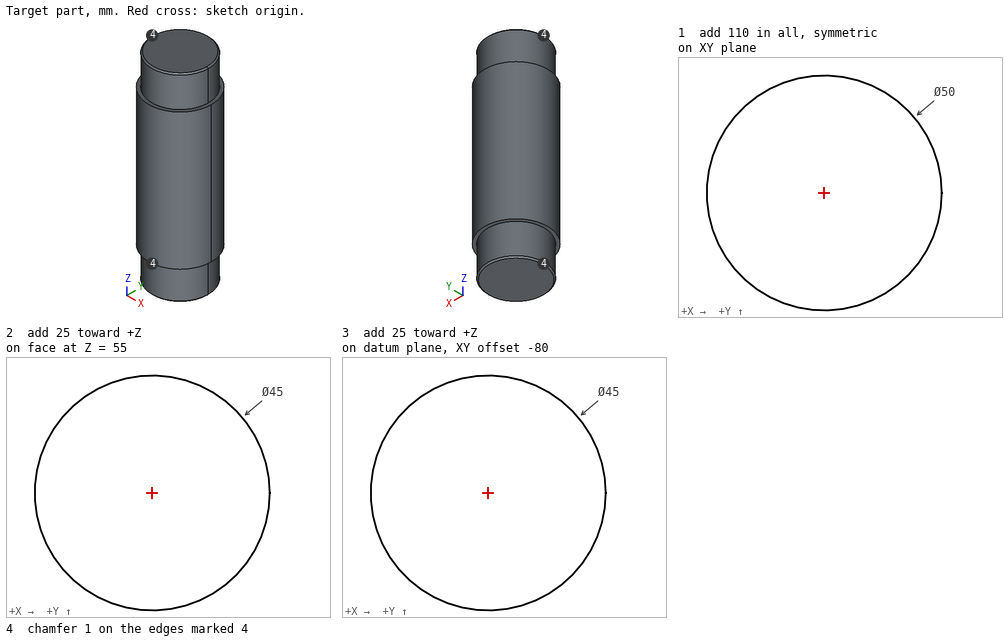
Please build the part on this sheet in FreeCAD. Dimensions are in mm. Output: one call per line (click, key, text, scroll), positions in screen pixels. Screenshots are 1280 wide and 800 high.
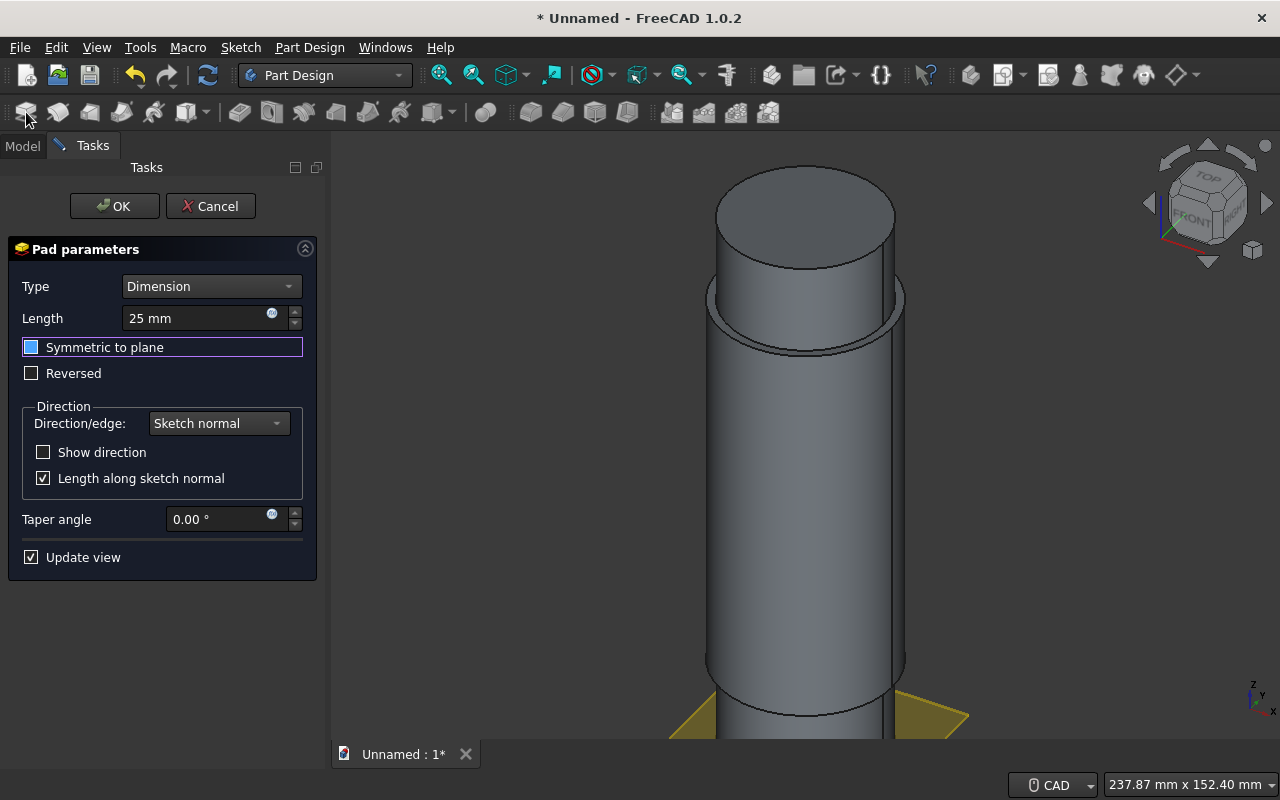
click(115, 206)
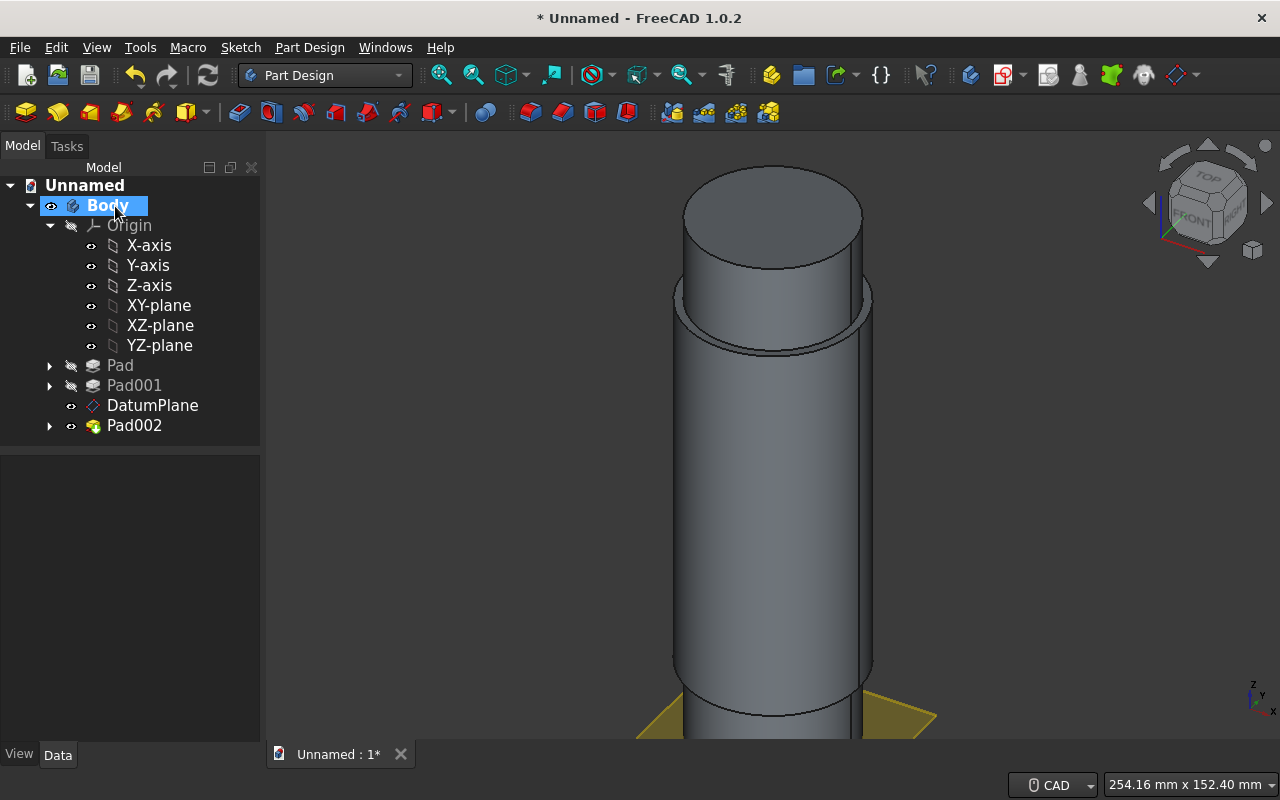
click(116, 406)
key(space)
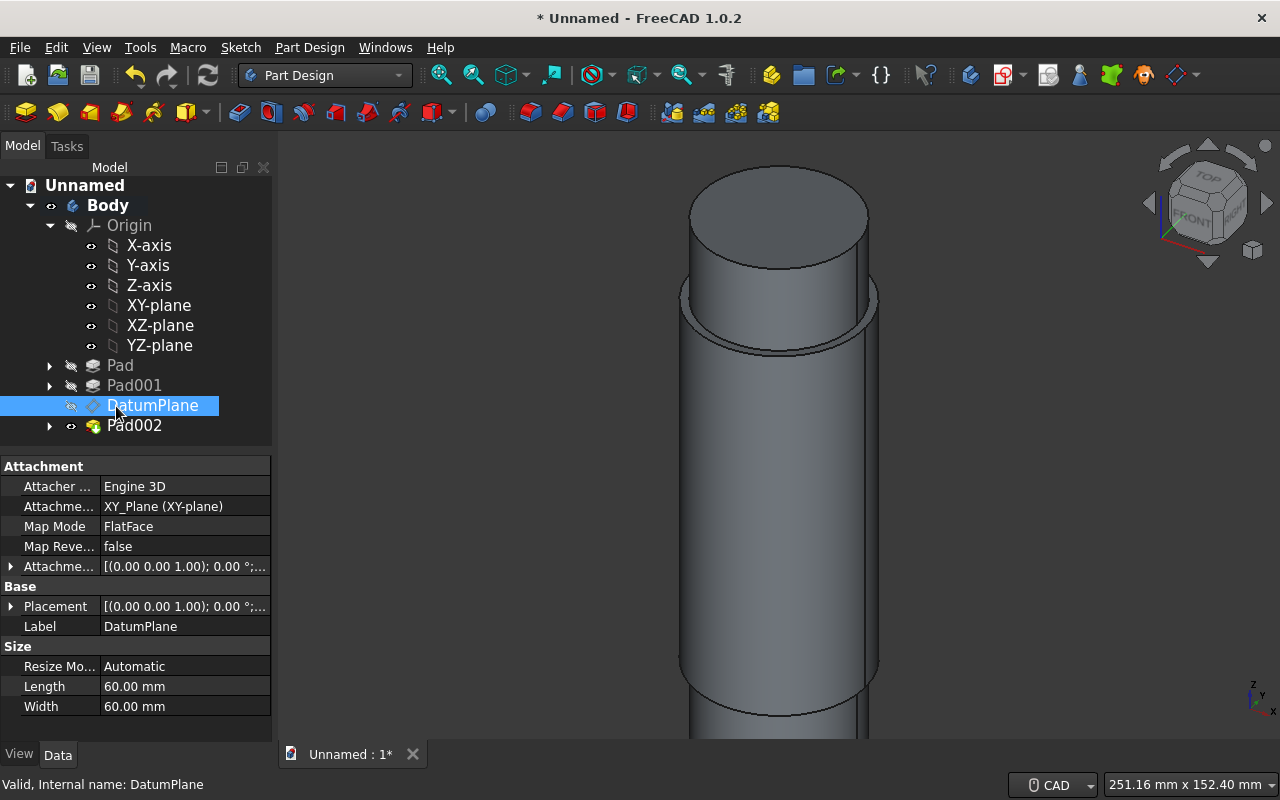
key(v)
key(f)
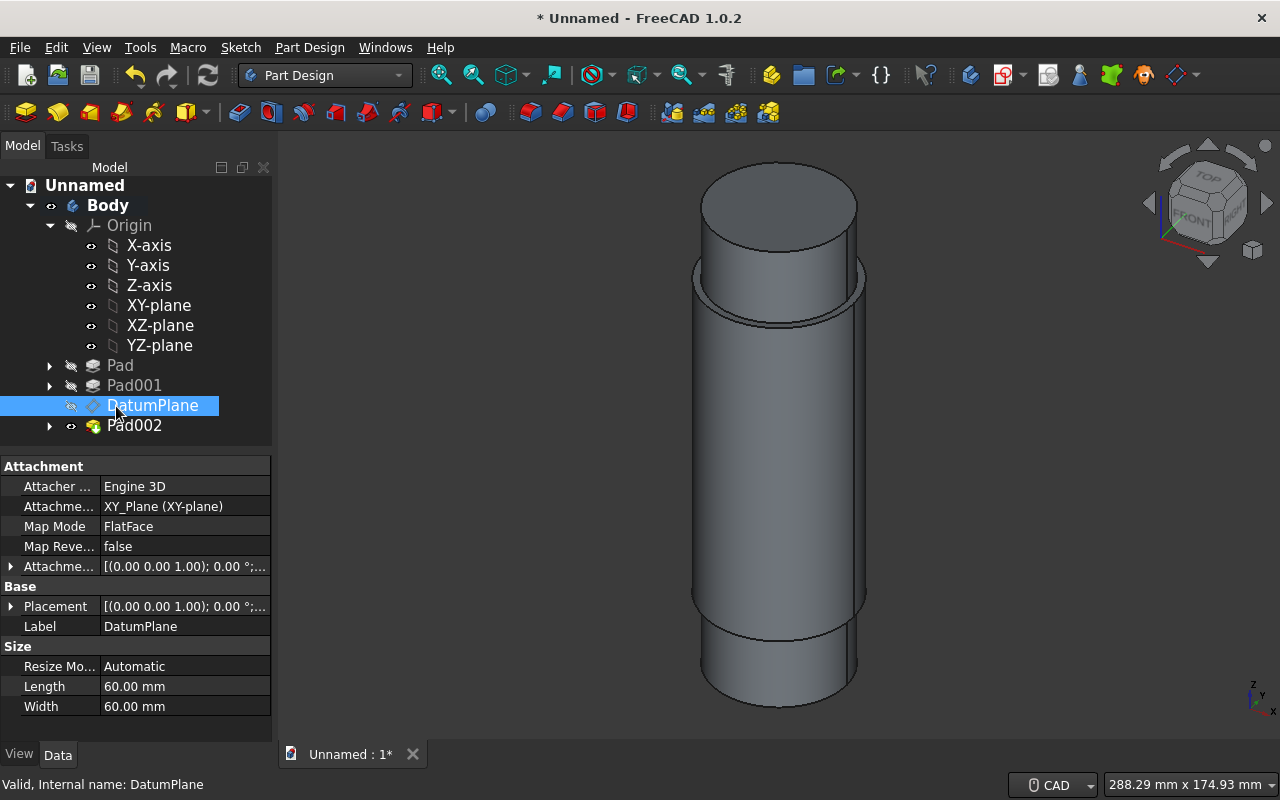
click(701, 211)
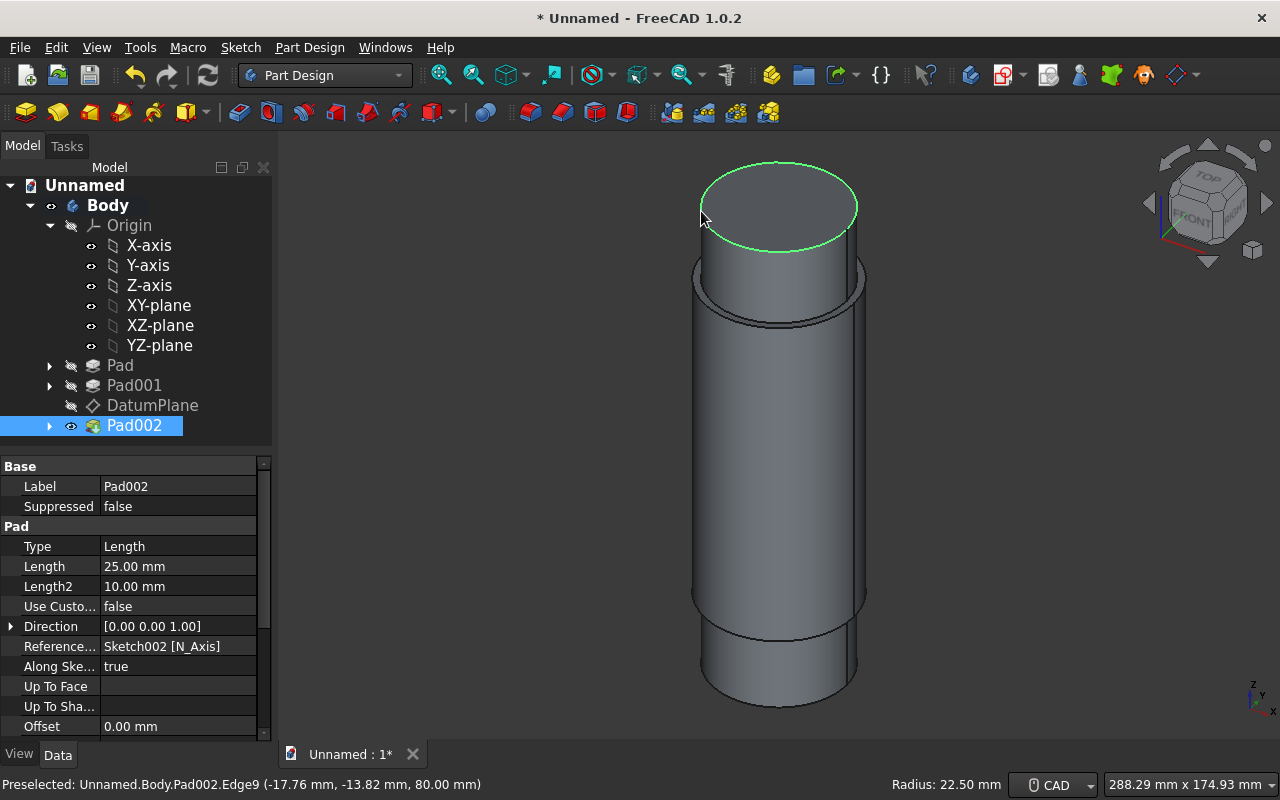
key(0)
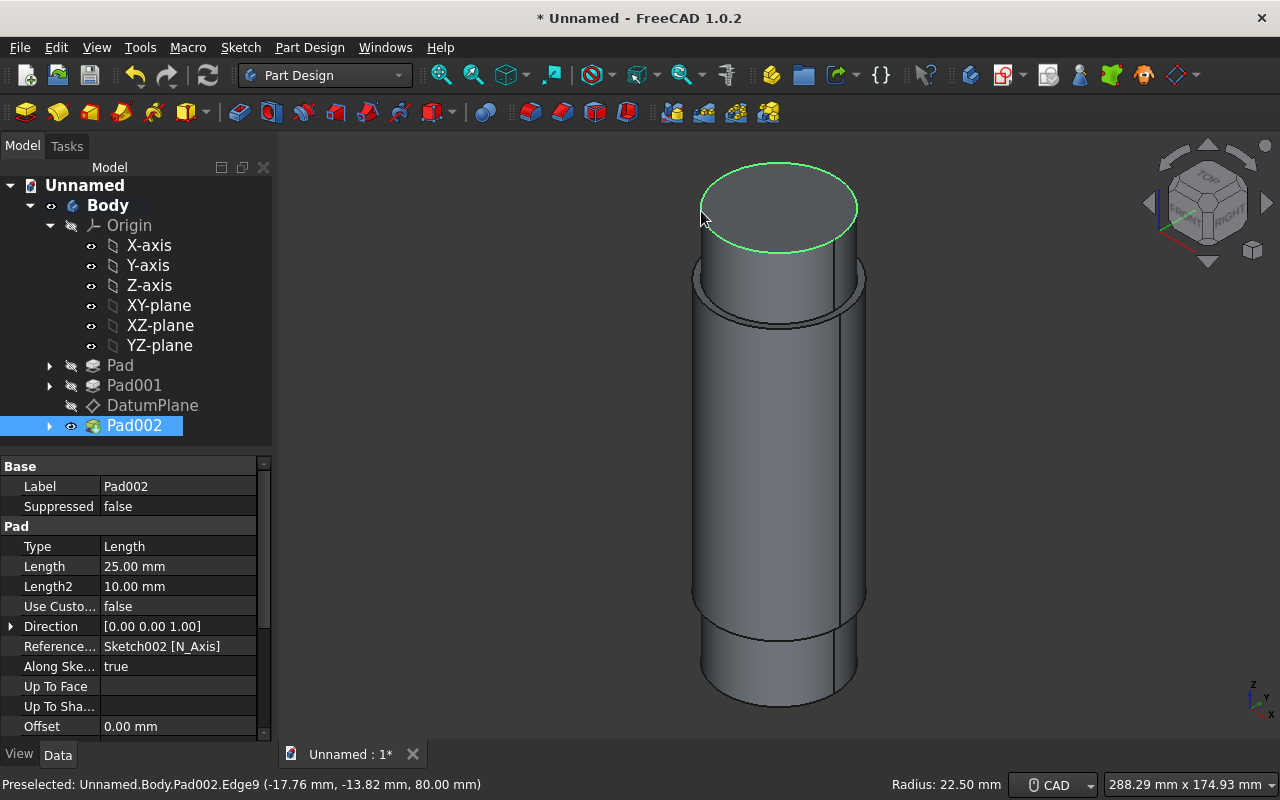
key(2)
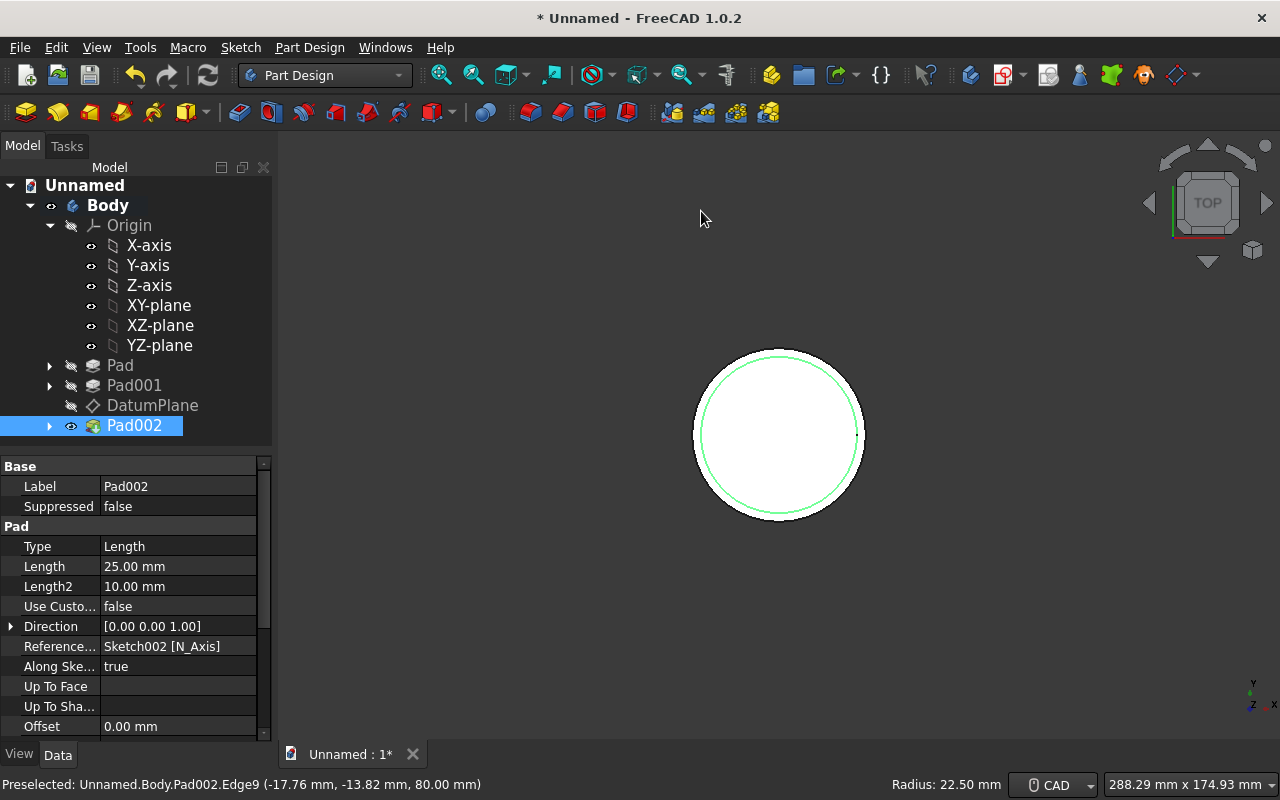
click(442, 76)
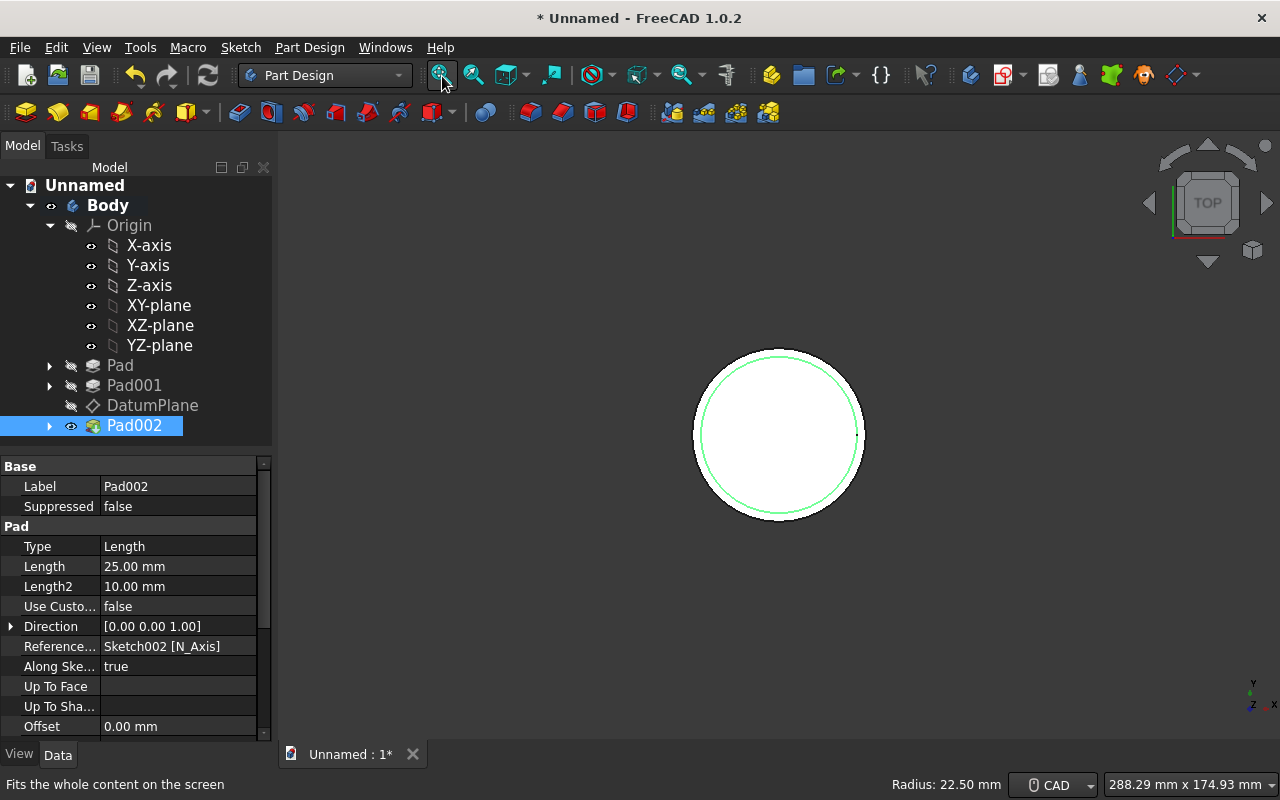
key(1)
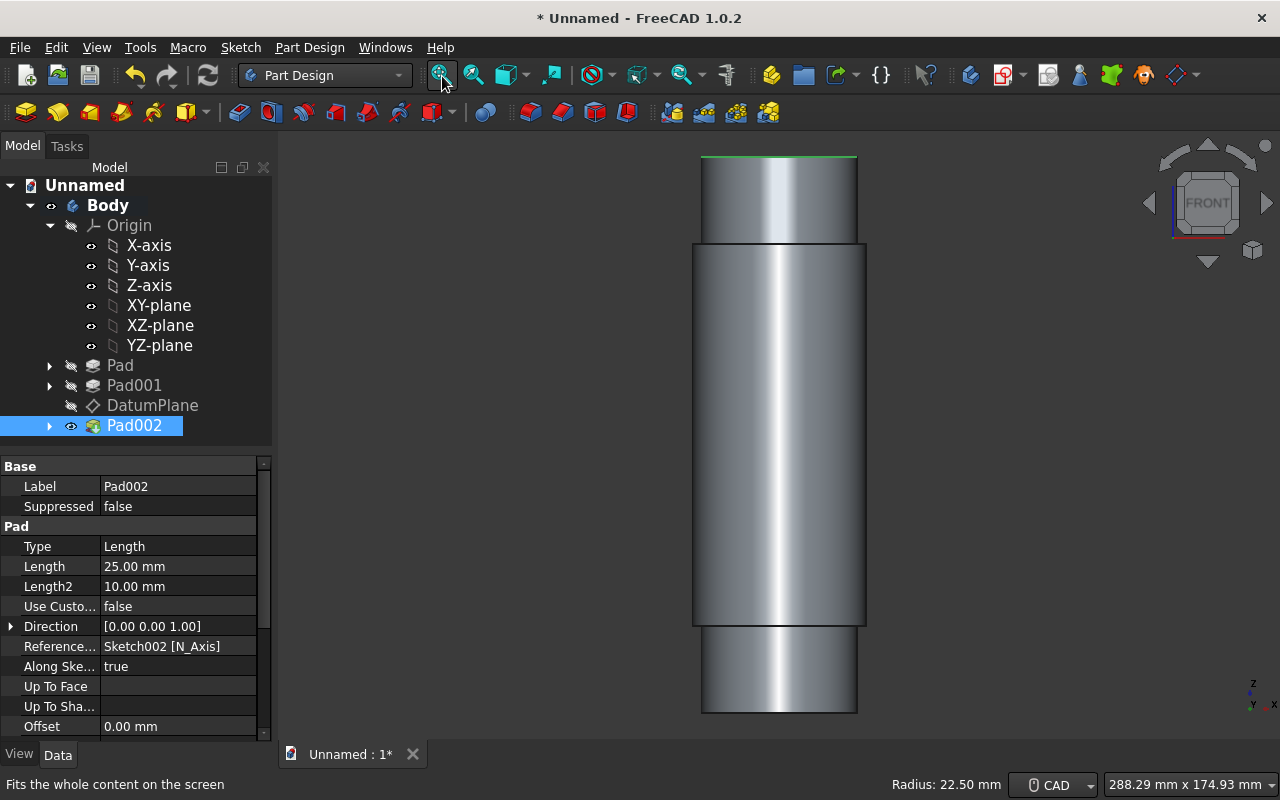
key(3)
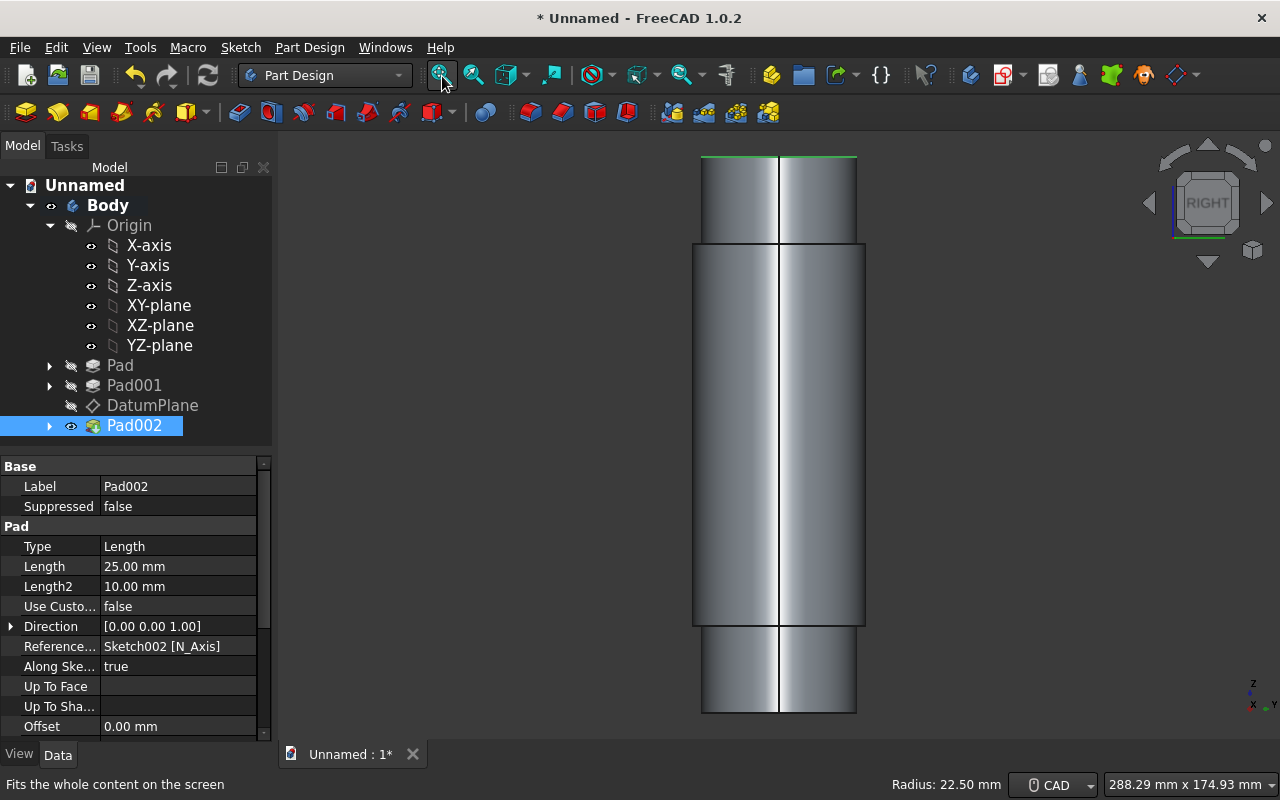
key(5)